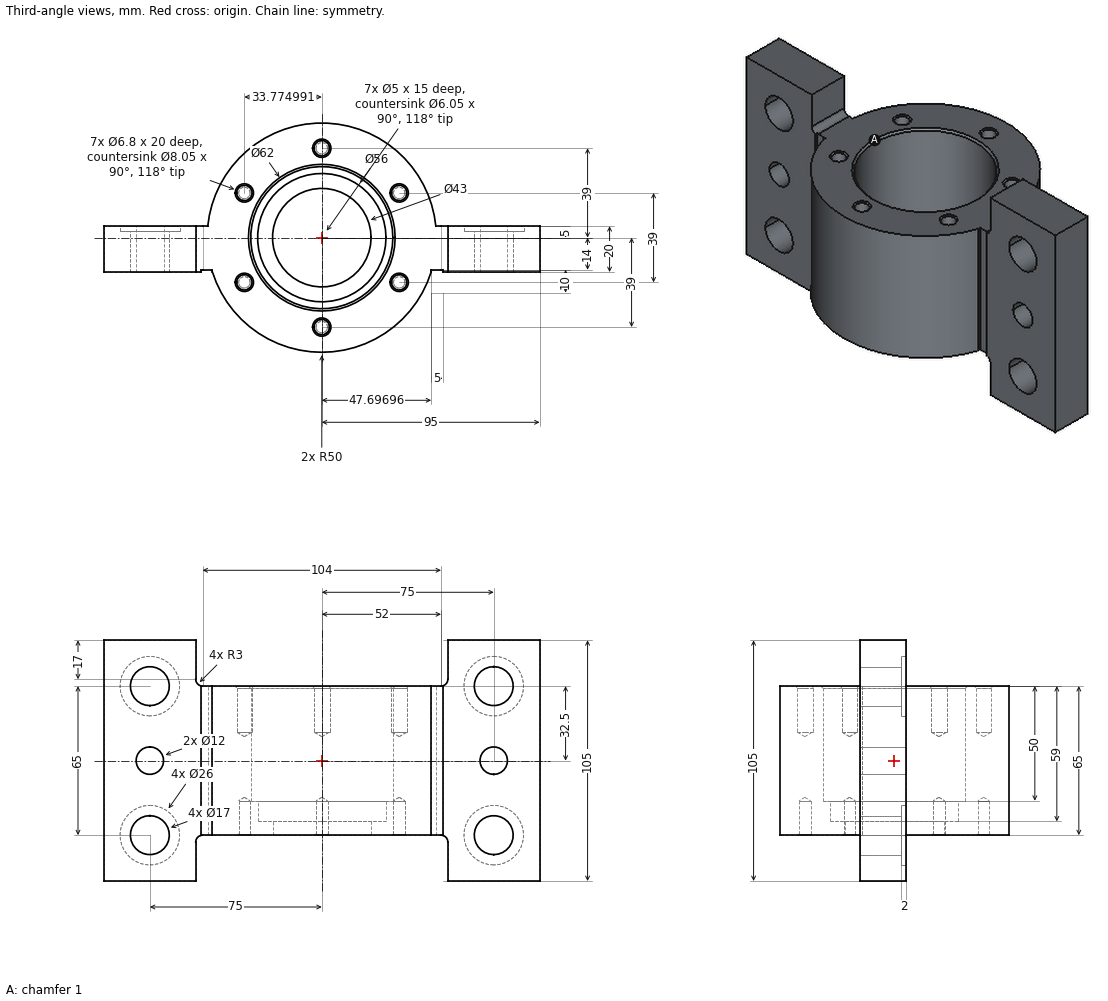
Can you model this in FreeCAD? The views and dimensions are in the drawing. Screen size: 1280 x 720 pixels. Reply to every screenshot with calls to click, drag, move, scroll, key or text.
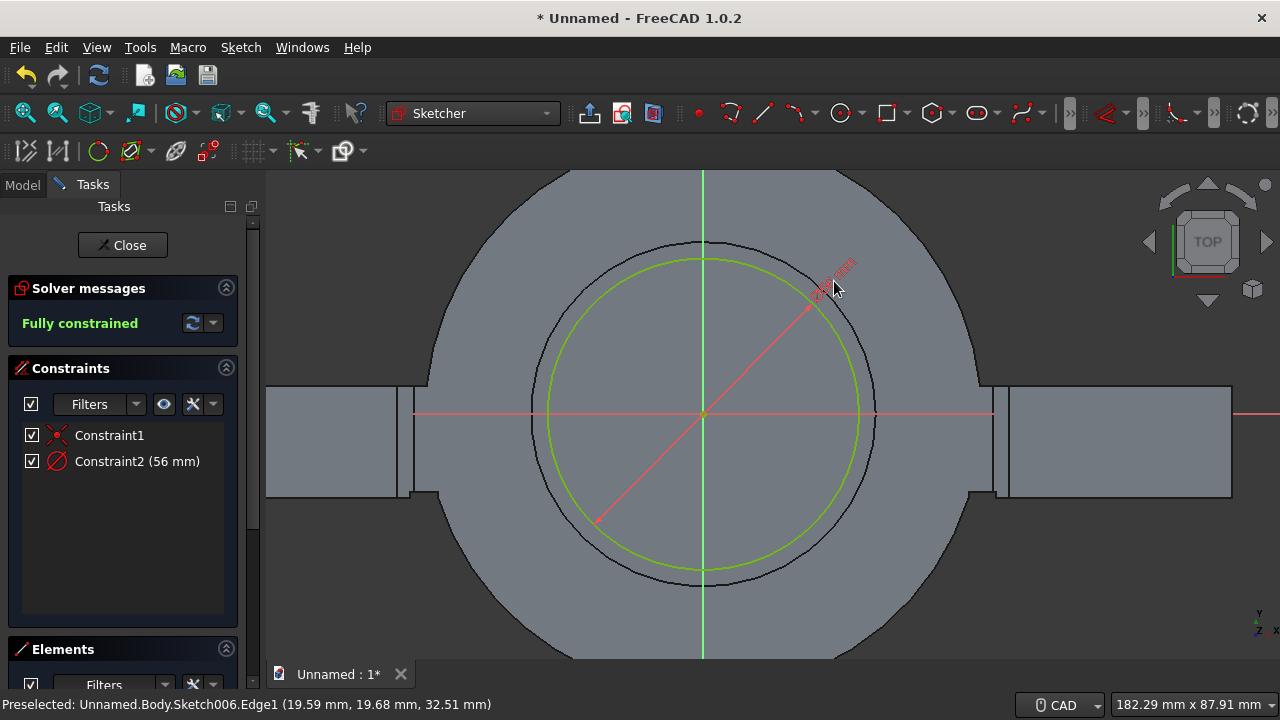
click(123, 245)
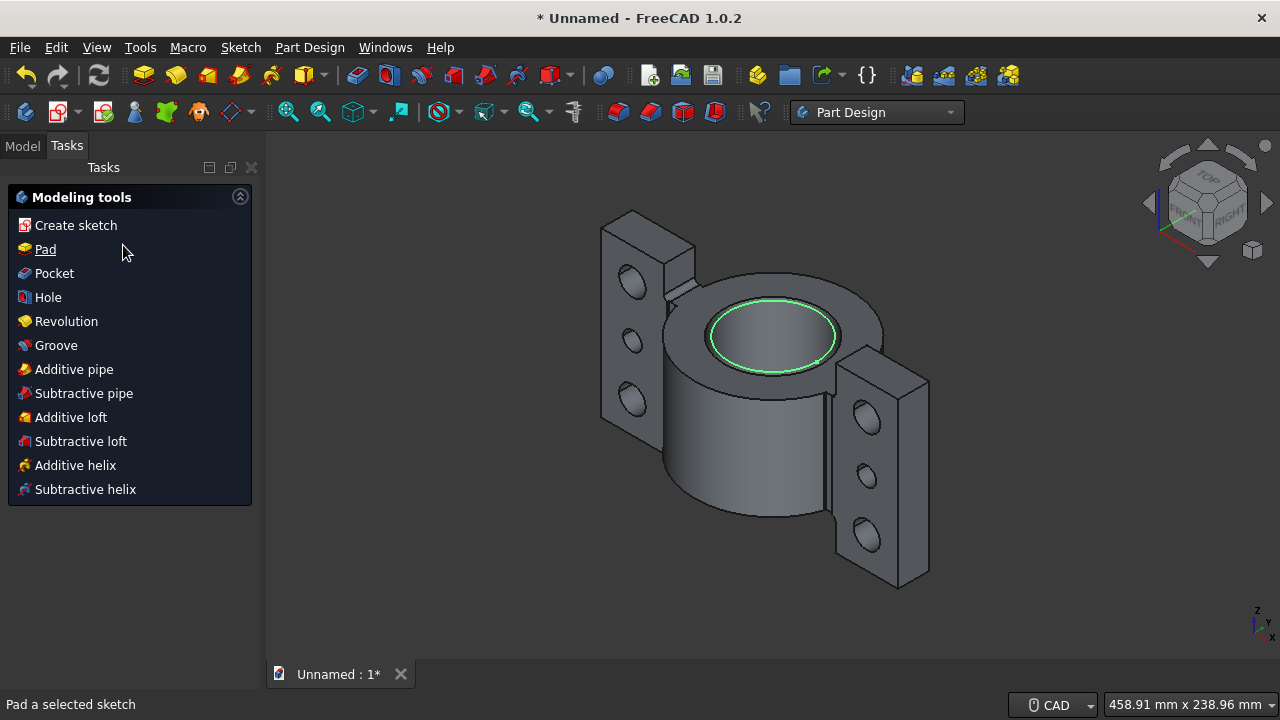
click(358, 76)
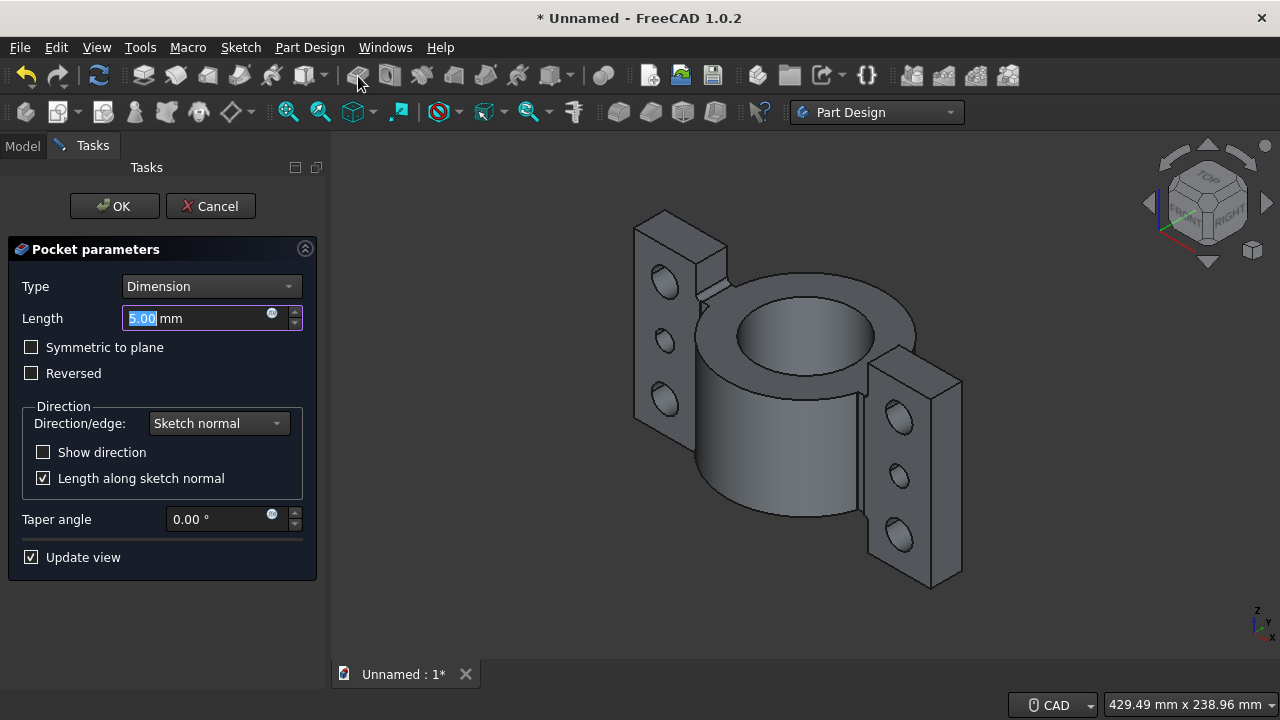
text(59)
key(Tab)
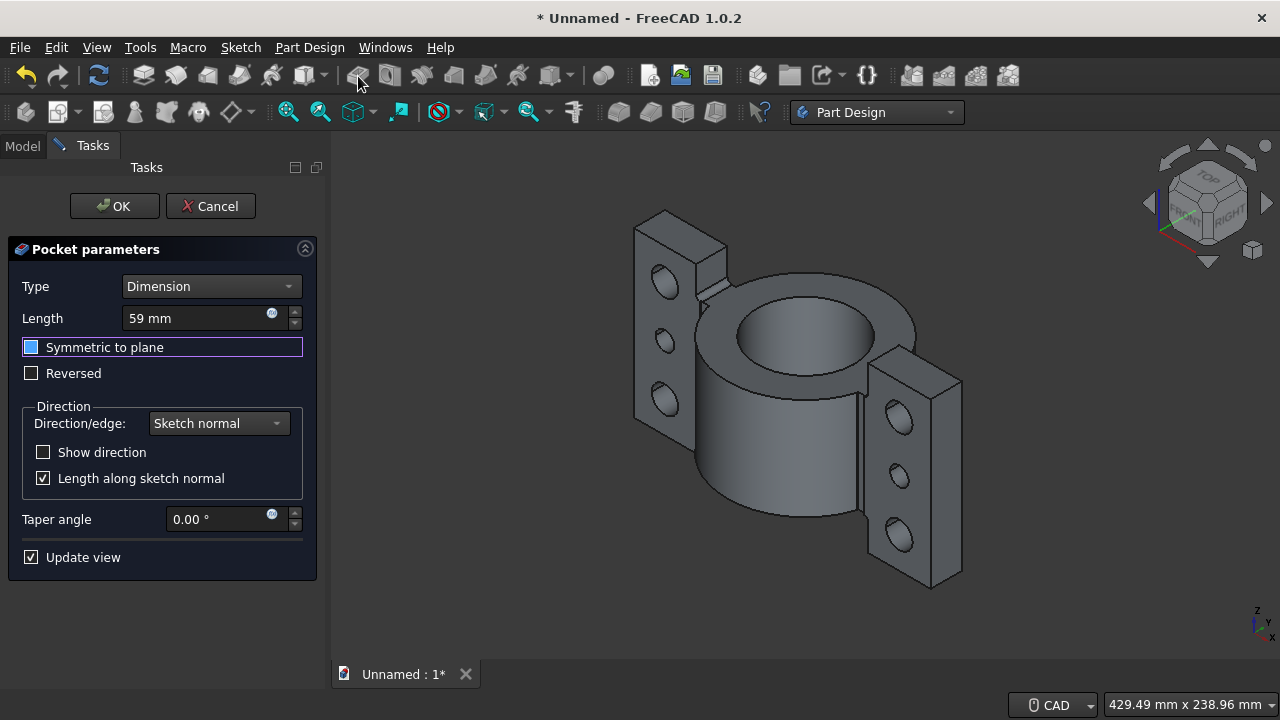
click(115, 206)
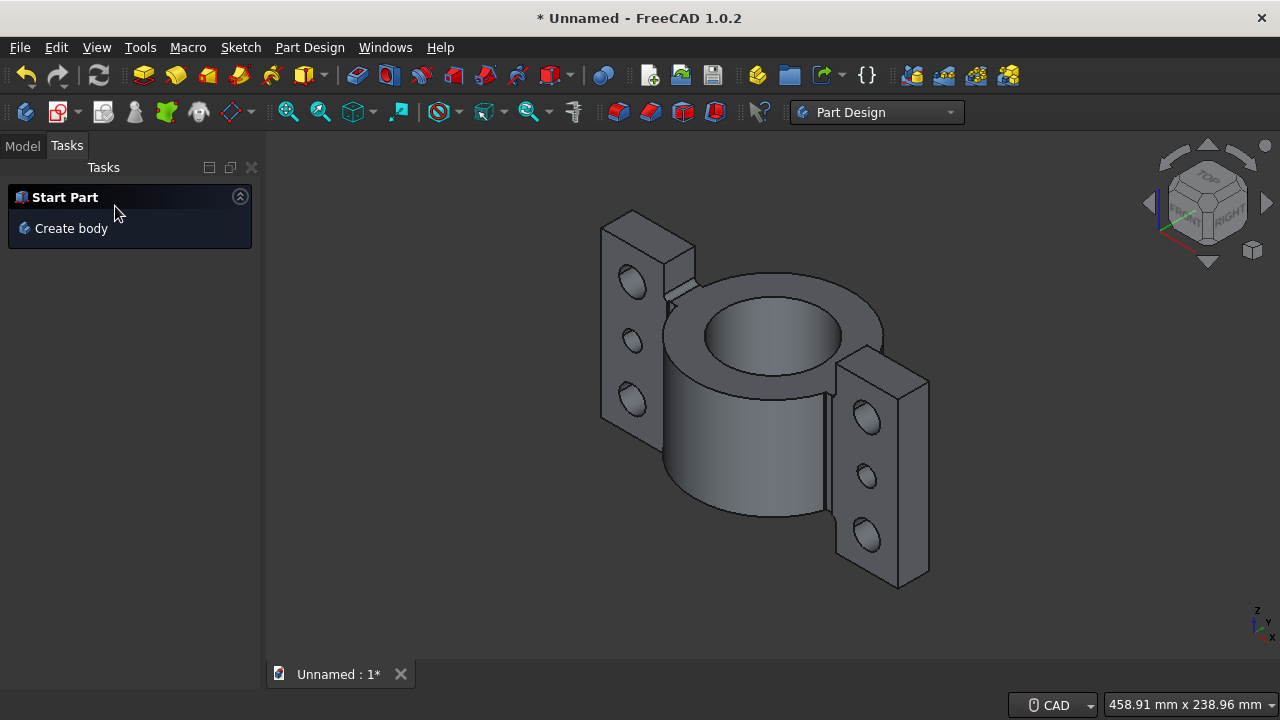
click(771, 283)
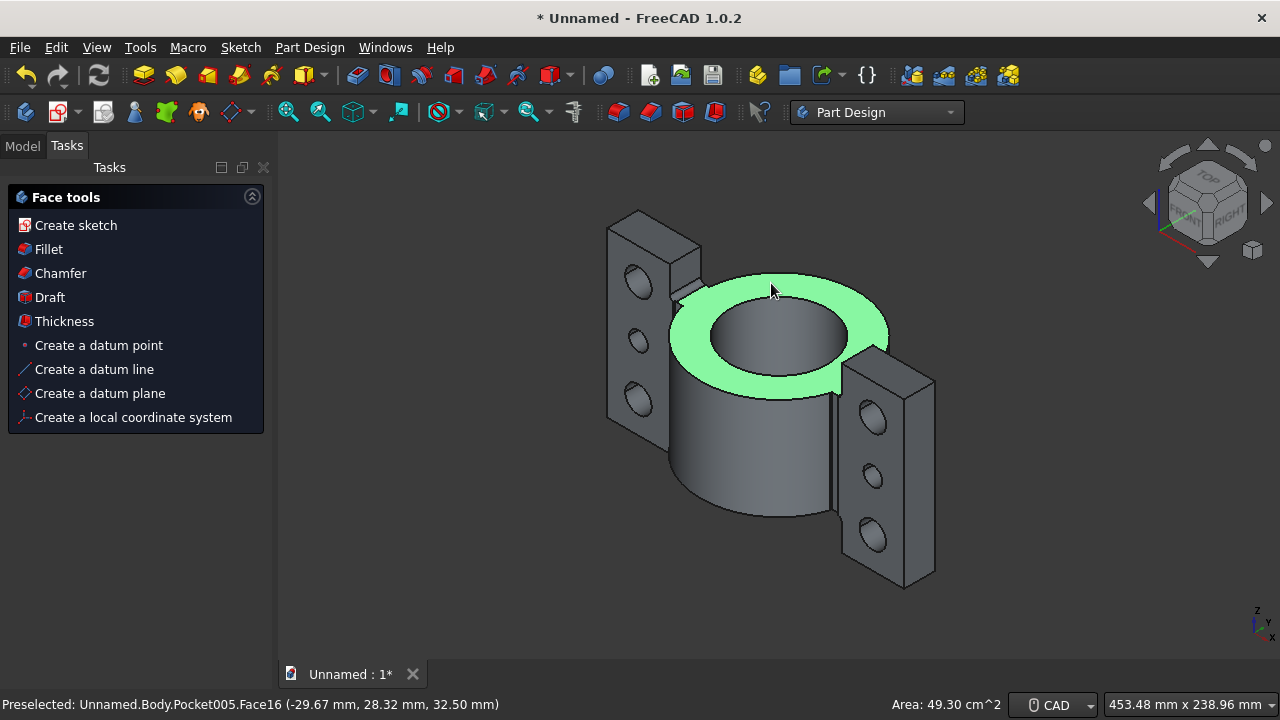
click(58, 112)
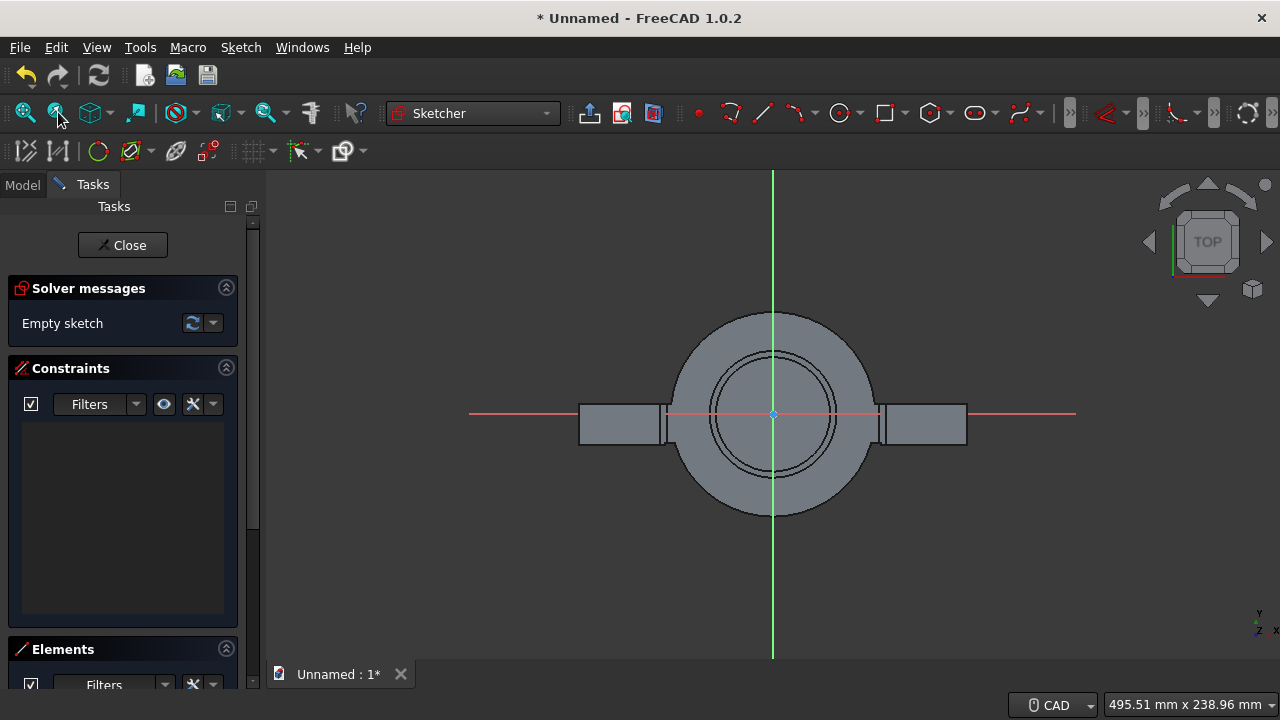
click(654, 114)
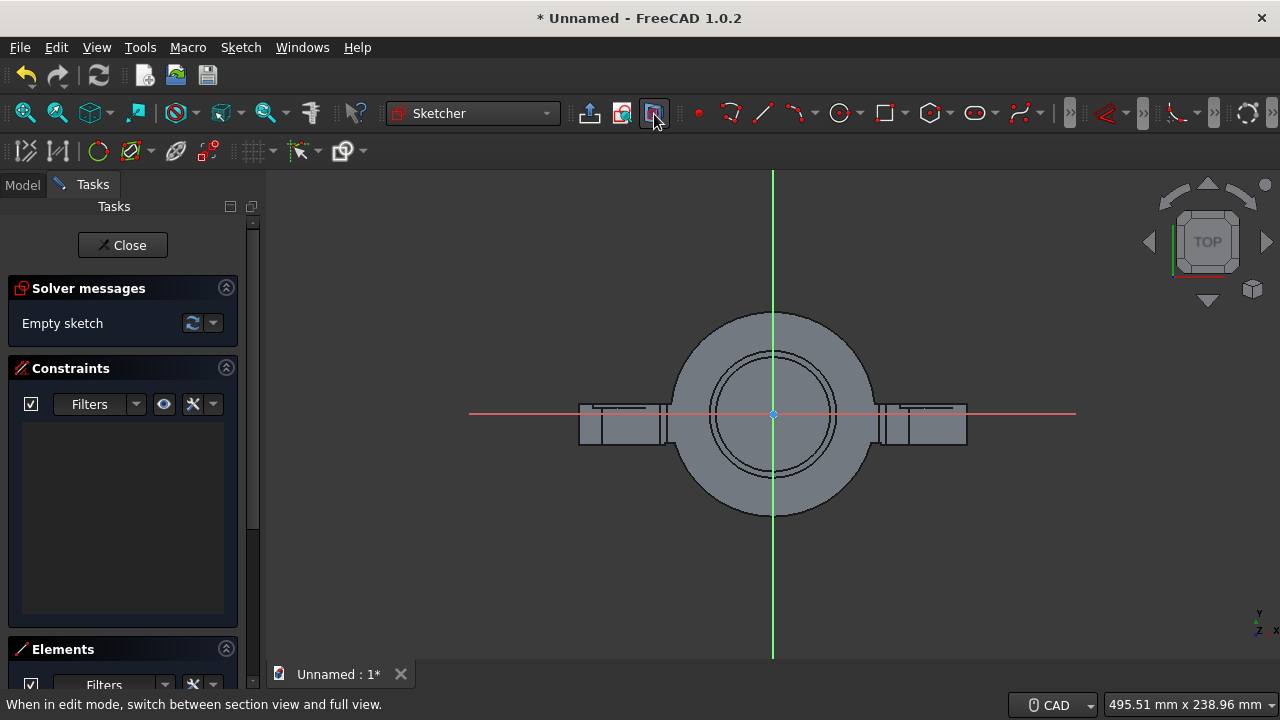
scroll(803, 414, up, 6)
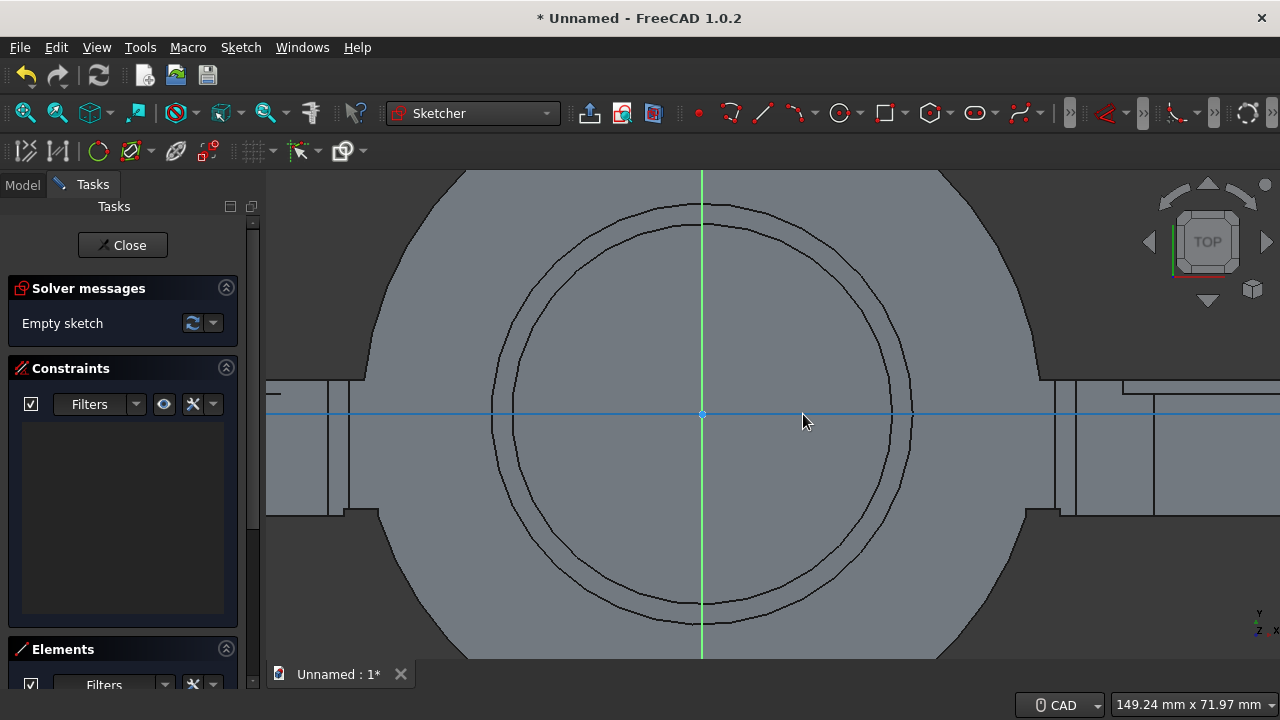
click(840, 114)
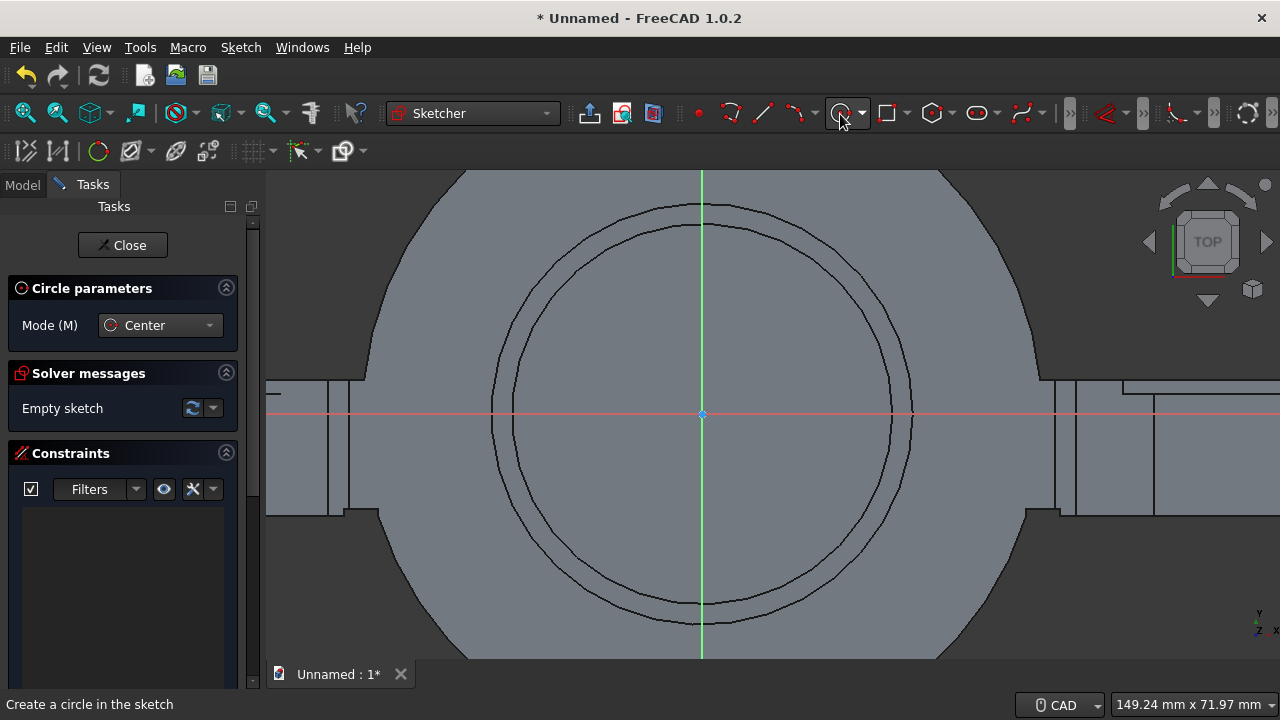
click(702, 414)
click(805, 311)
key(Escape)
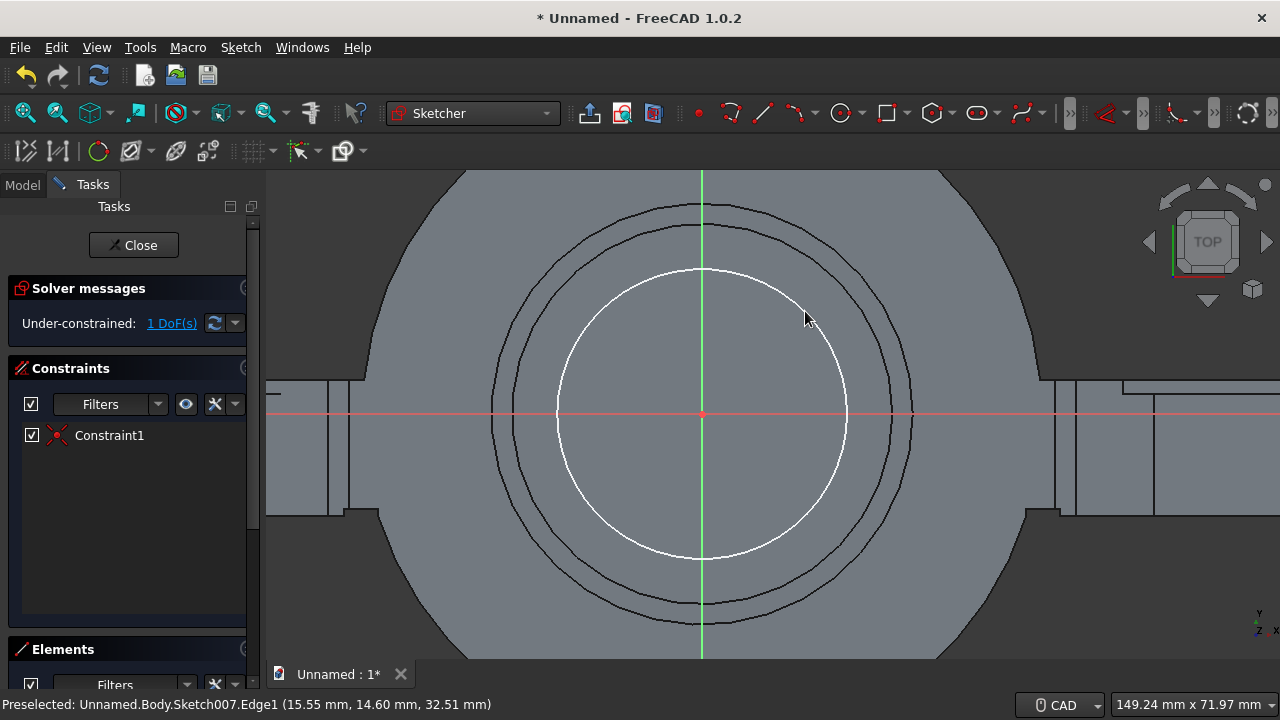
click(1106, 114)